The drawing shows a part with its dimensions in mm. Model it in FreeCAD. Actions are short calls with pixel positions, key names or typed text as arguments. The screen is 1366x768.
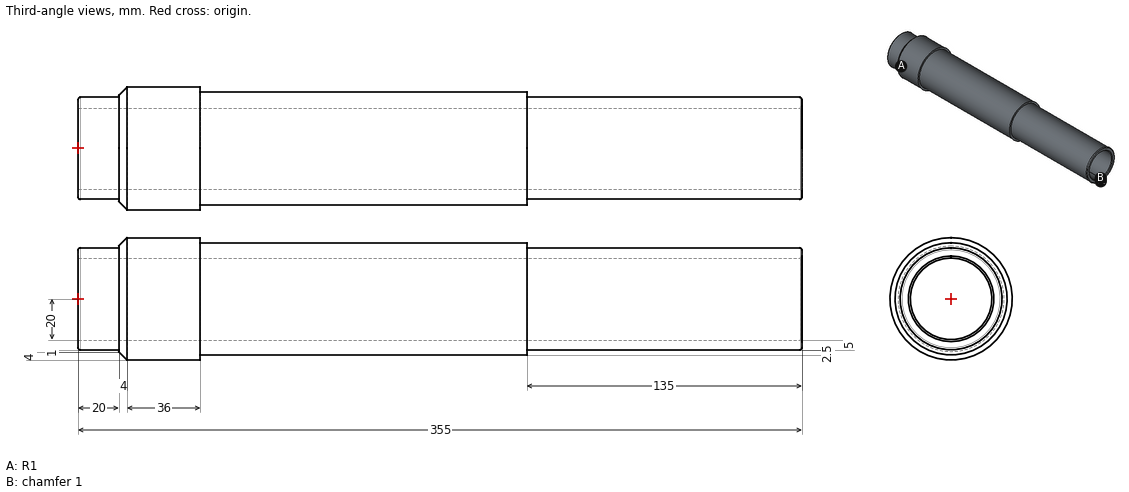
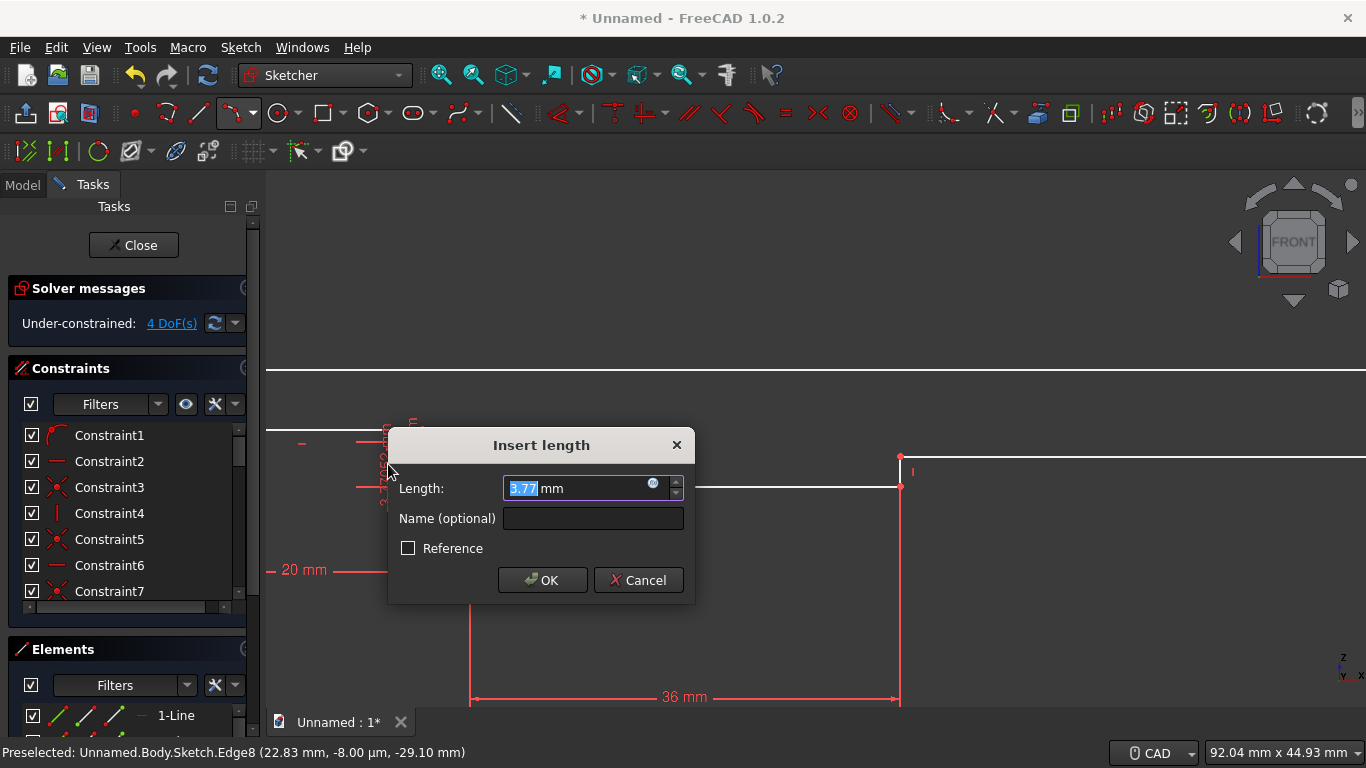
text(4)
key(Return)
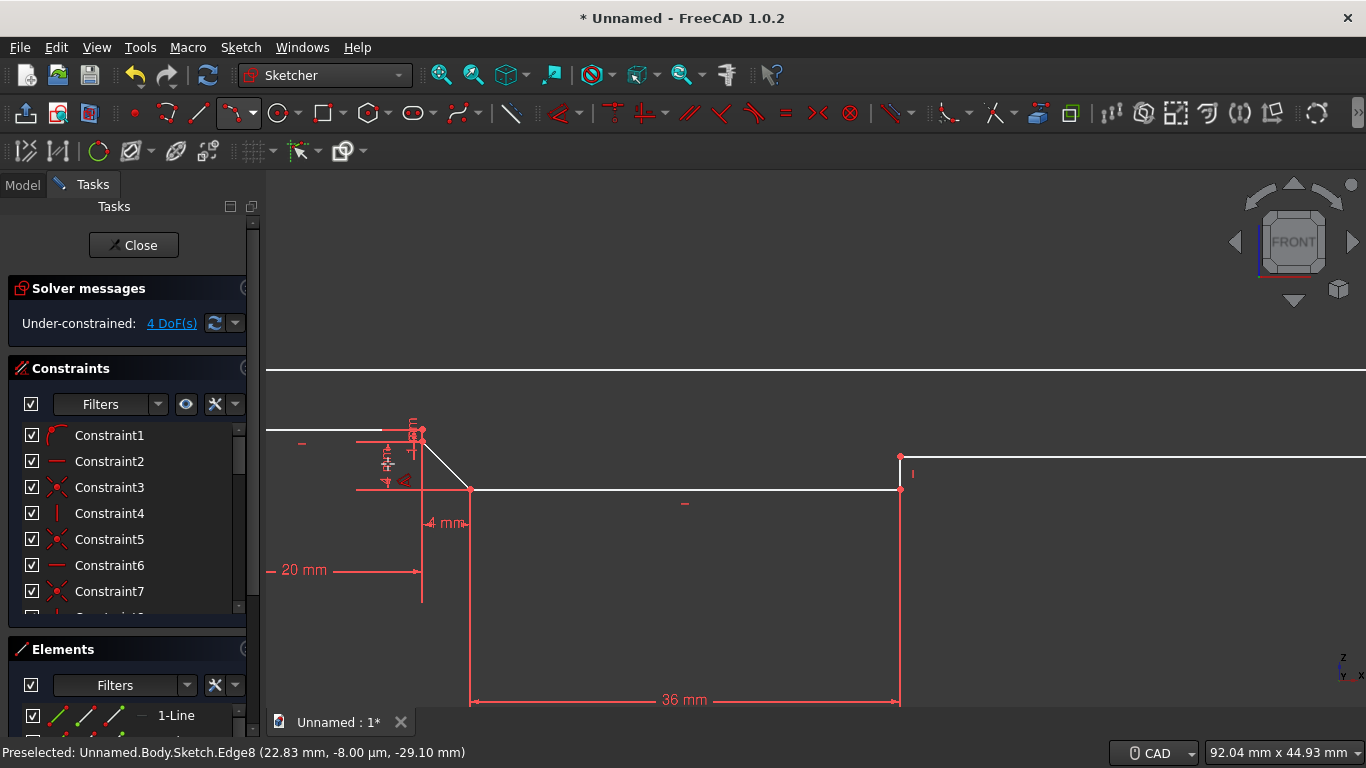
scroll(439, 465, down, 9)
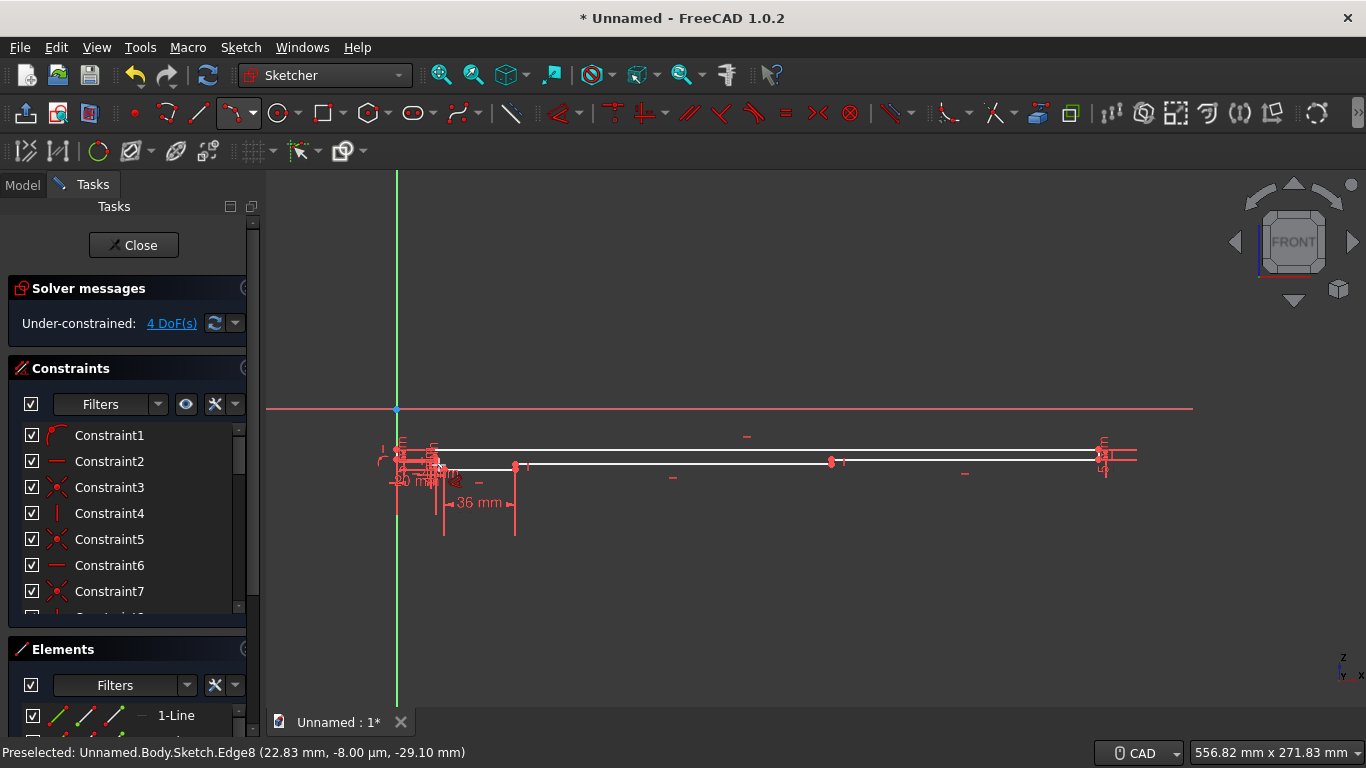
click(537, 450)
click(748, 484)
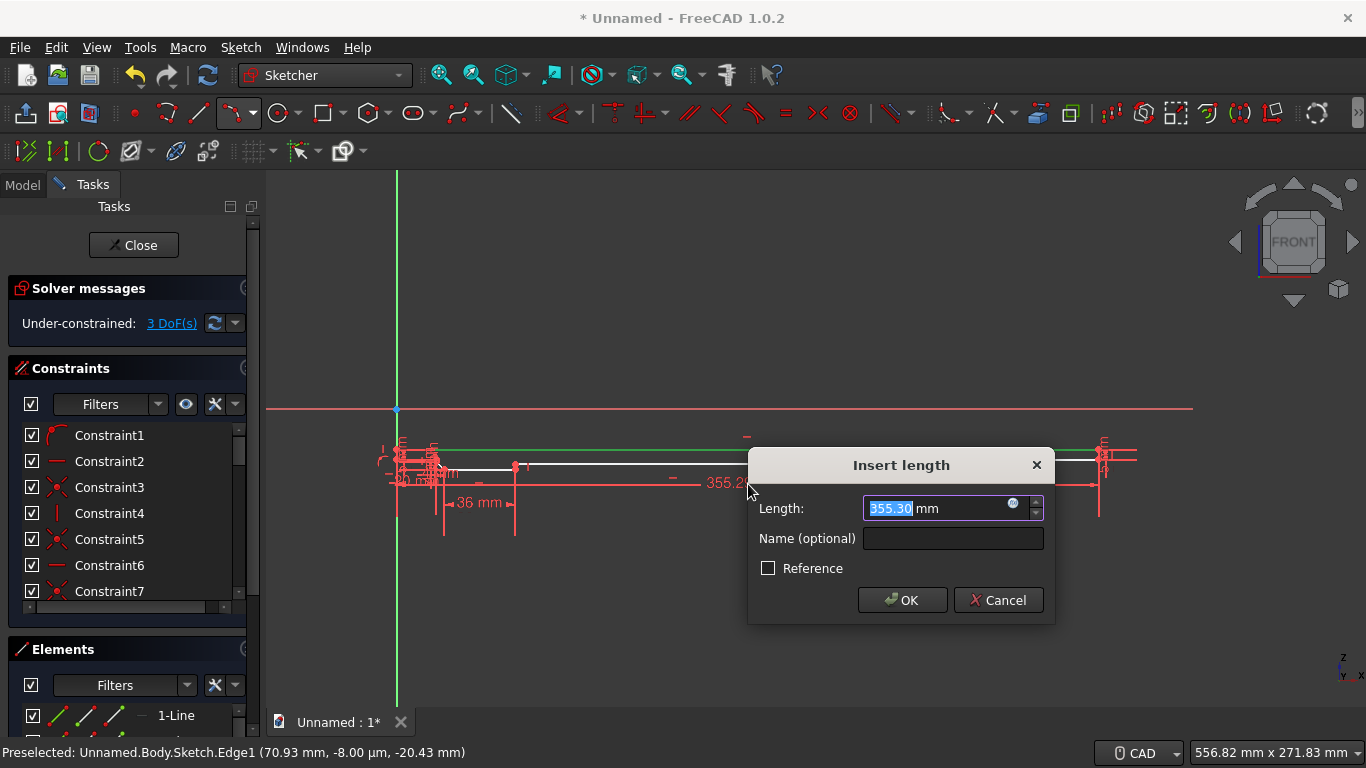
text(355)
key(Return)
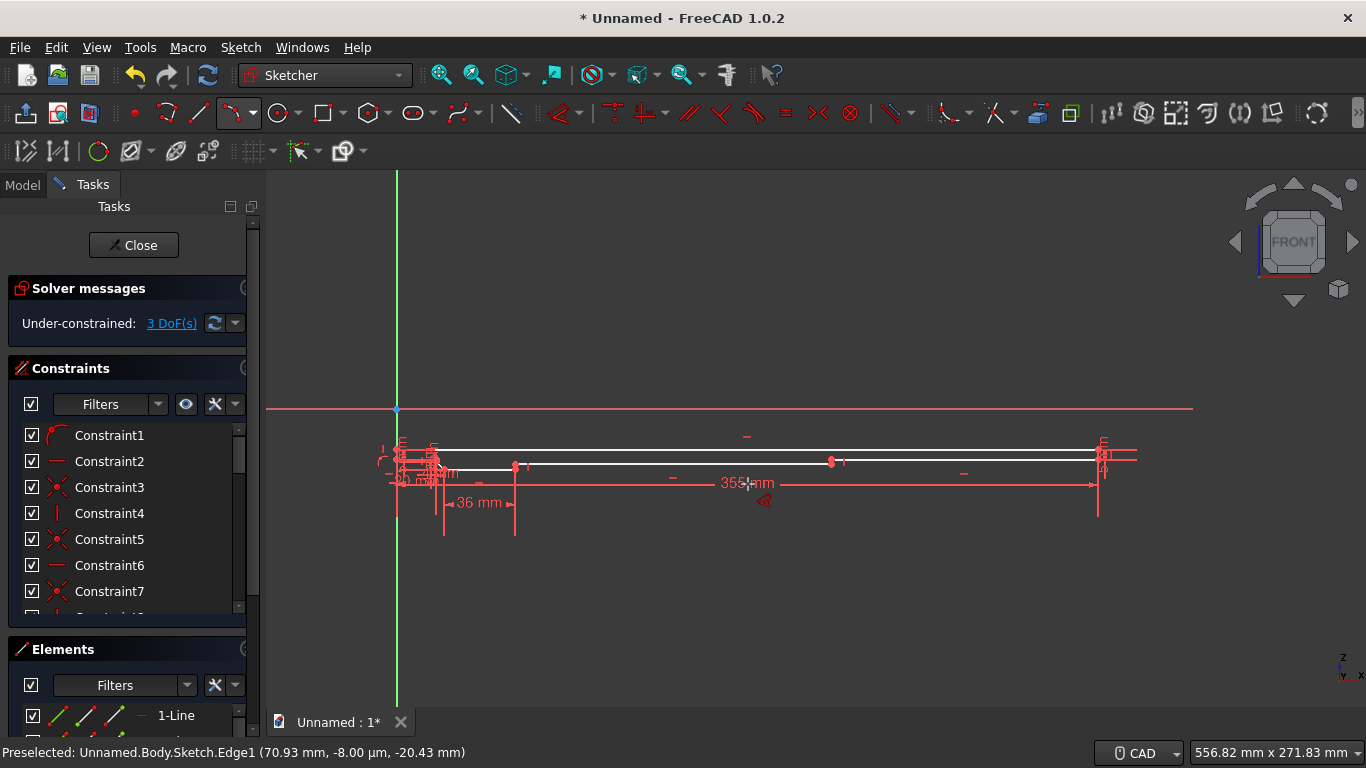
scroll(1018, 460, up, 2)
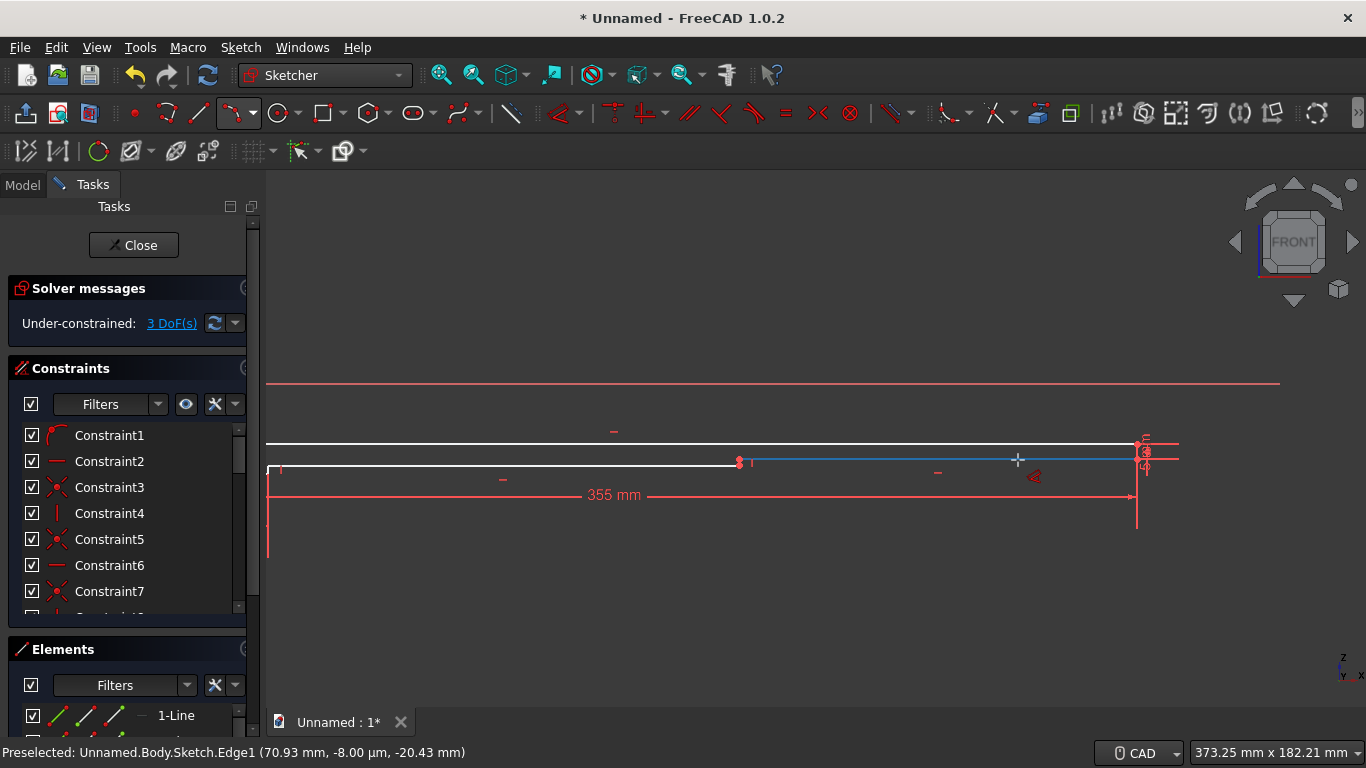
click(1018, 459)
click(938, 493)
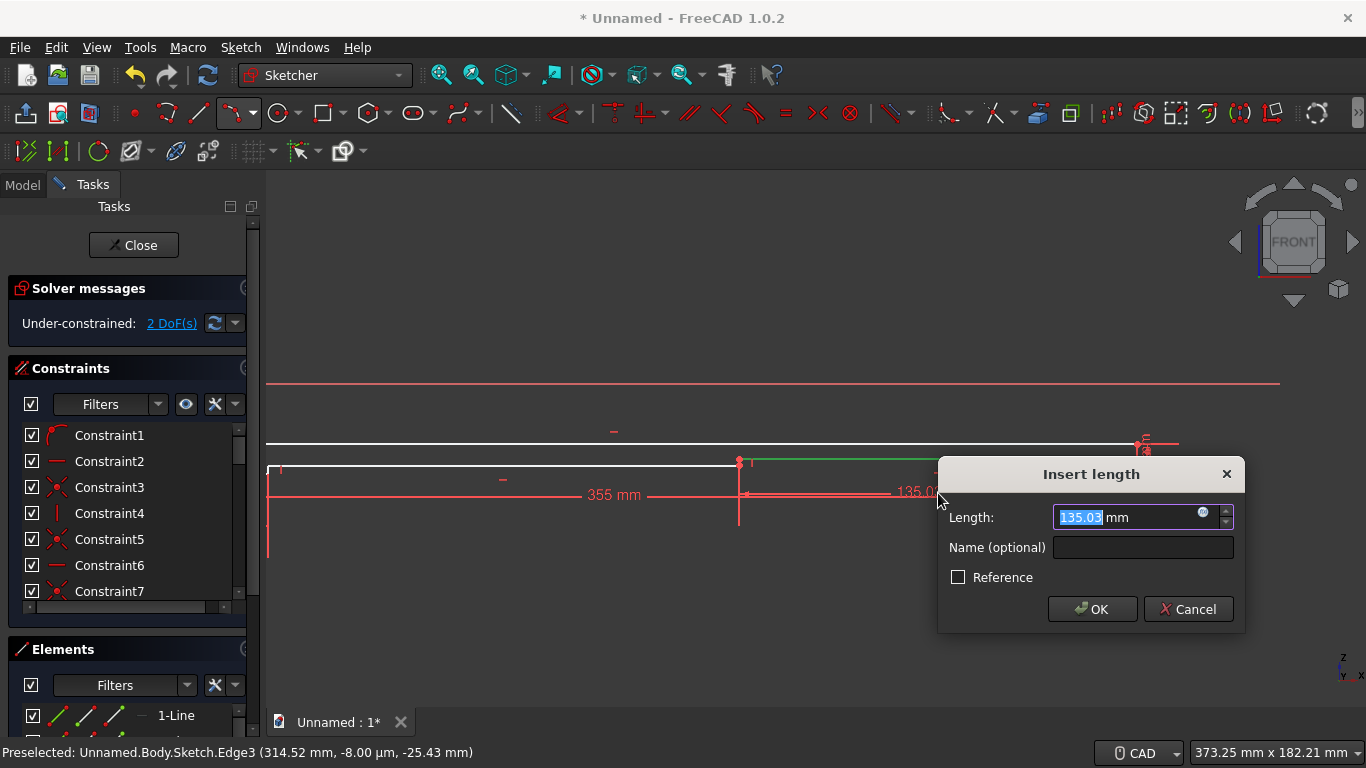
text(135)
key(Return)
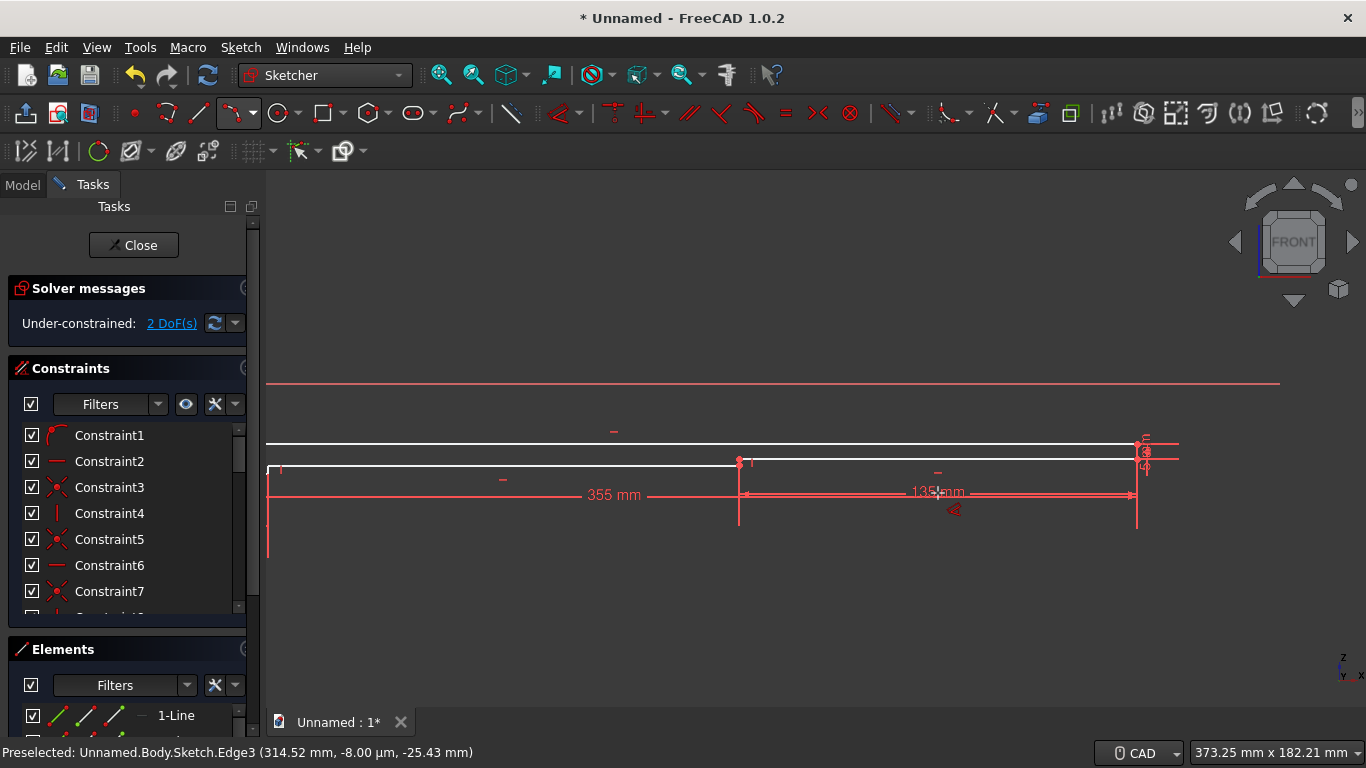
scroll(739, 463, up, 9)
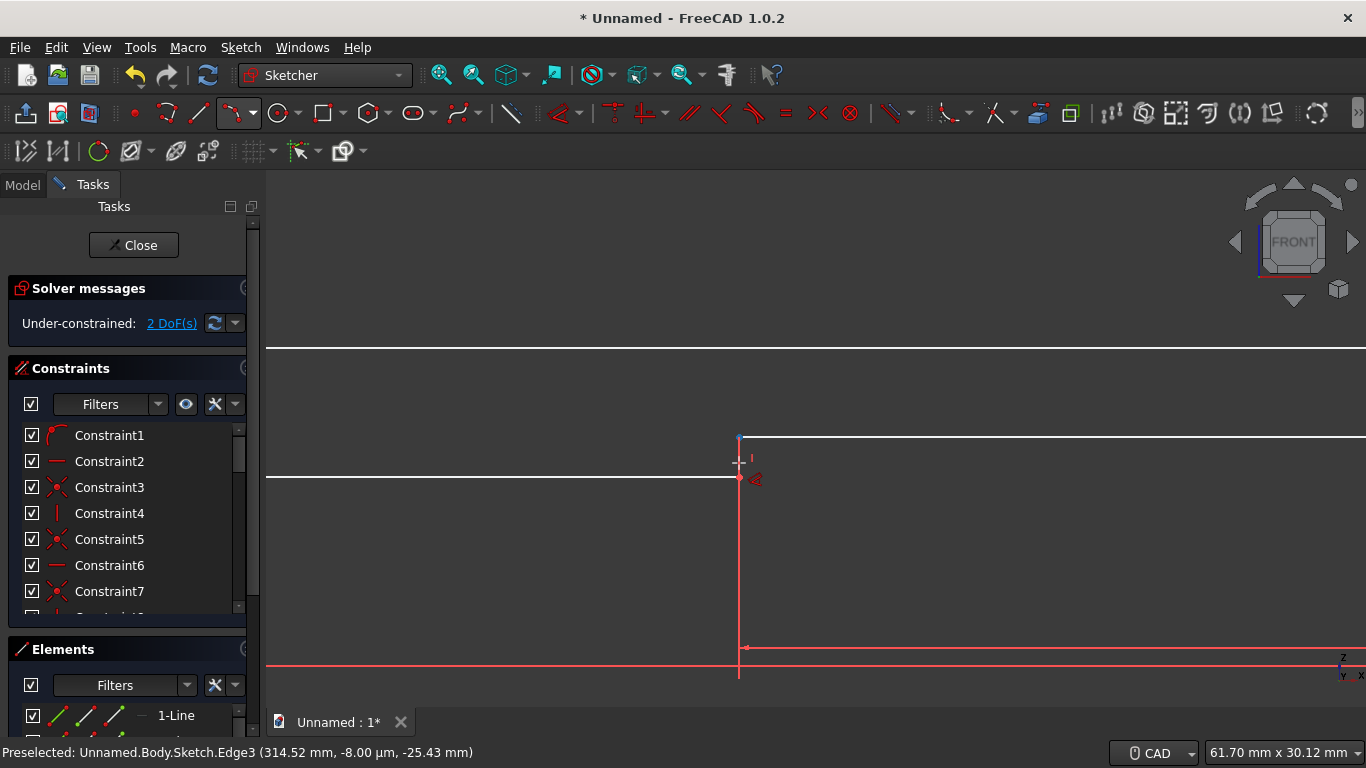
click(739, 457)
click(773, 457)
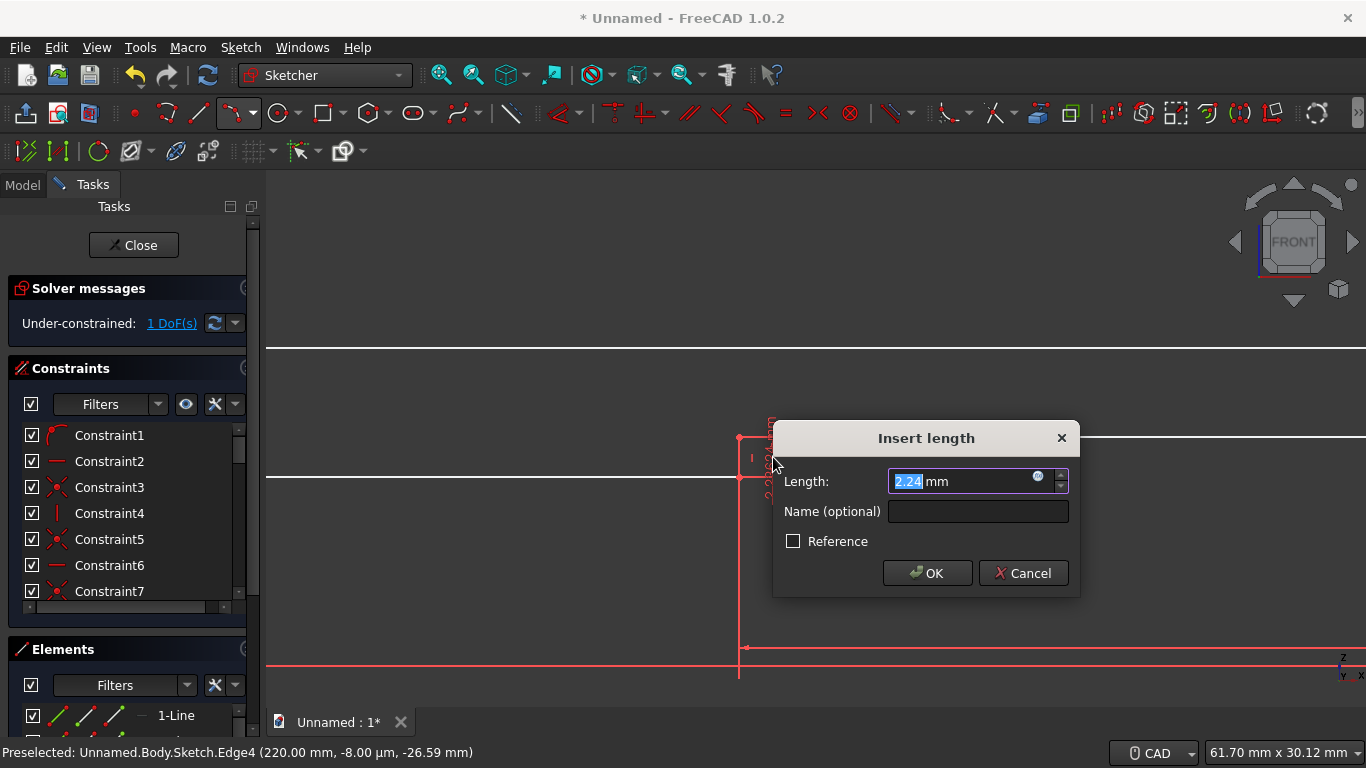
text(2.5)
key(Return)